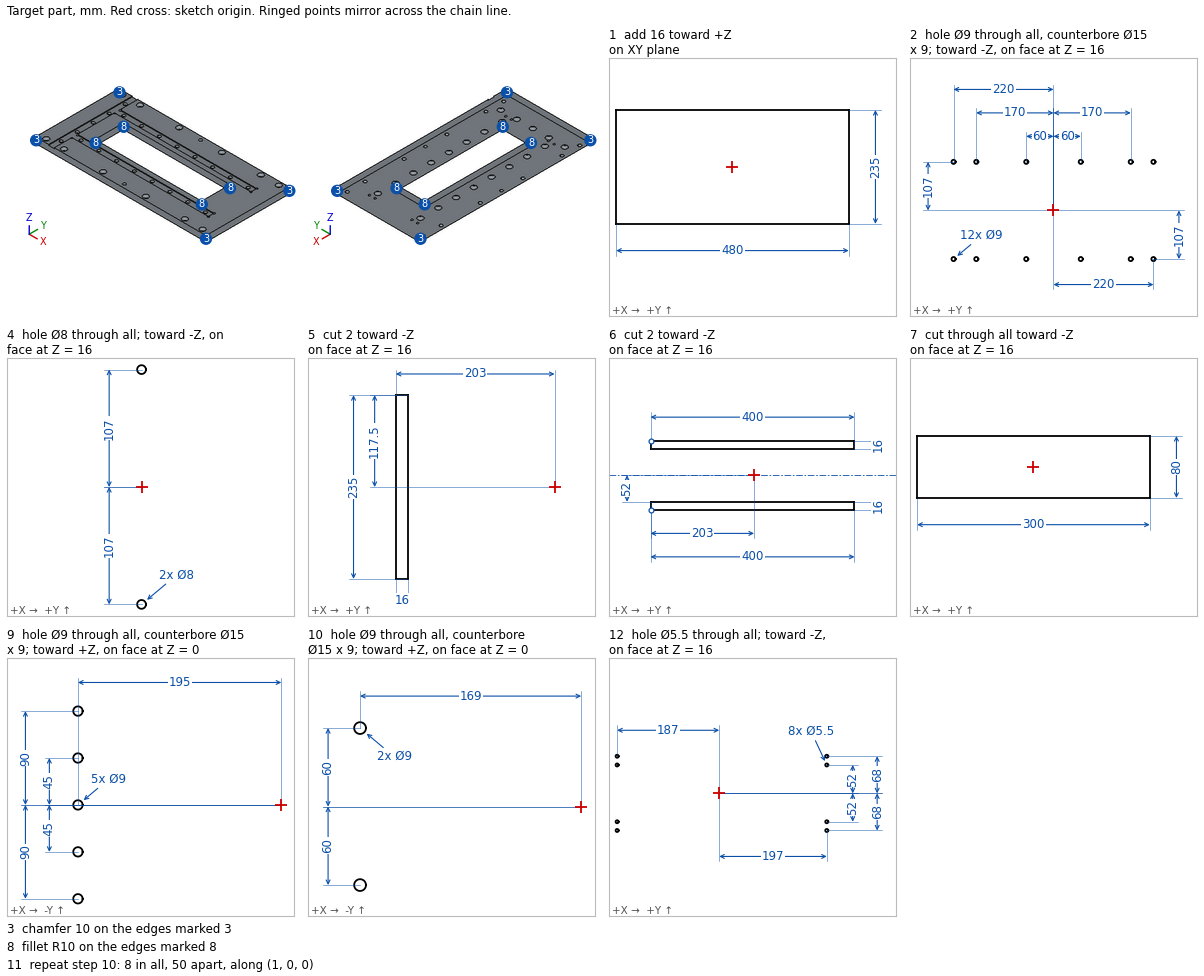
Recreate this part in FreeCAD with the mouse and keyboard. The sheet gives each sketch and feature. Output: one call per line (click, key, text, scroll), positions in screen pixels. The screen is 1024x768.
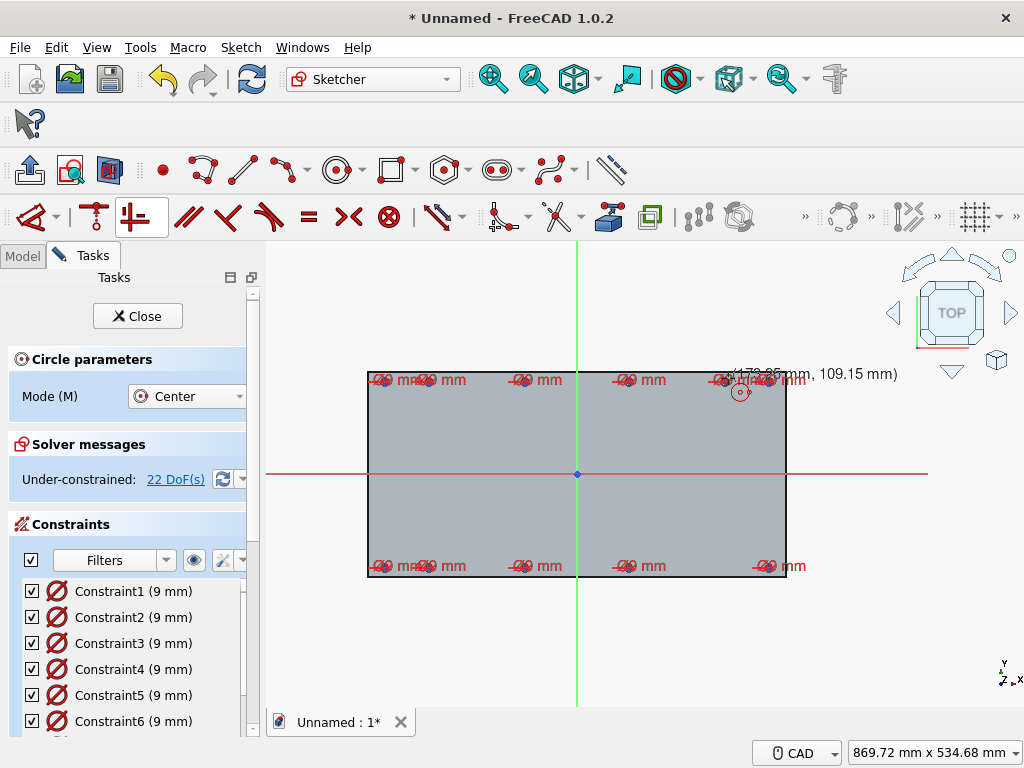
scroll(725, 567, up, 9)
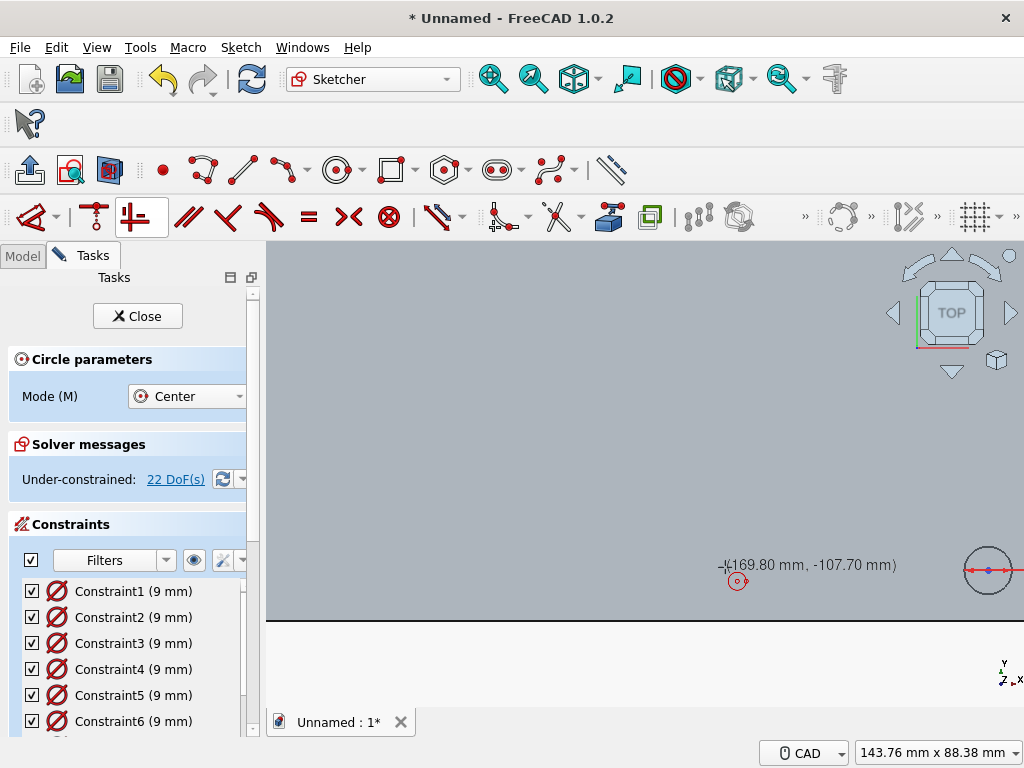
scroll(725, 568, down, 9)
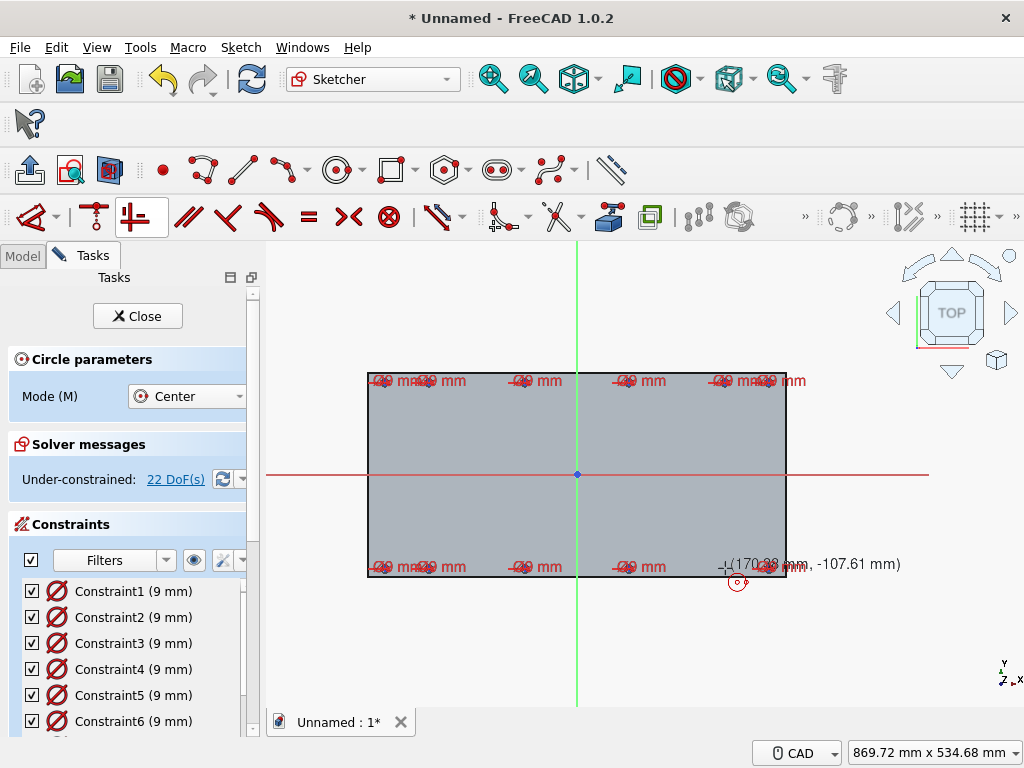
click(725, 568)
move(728, 565)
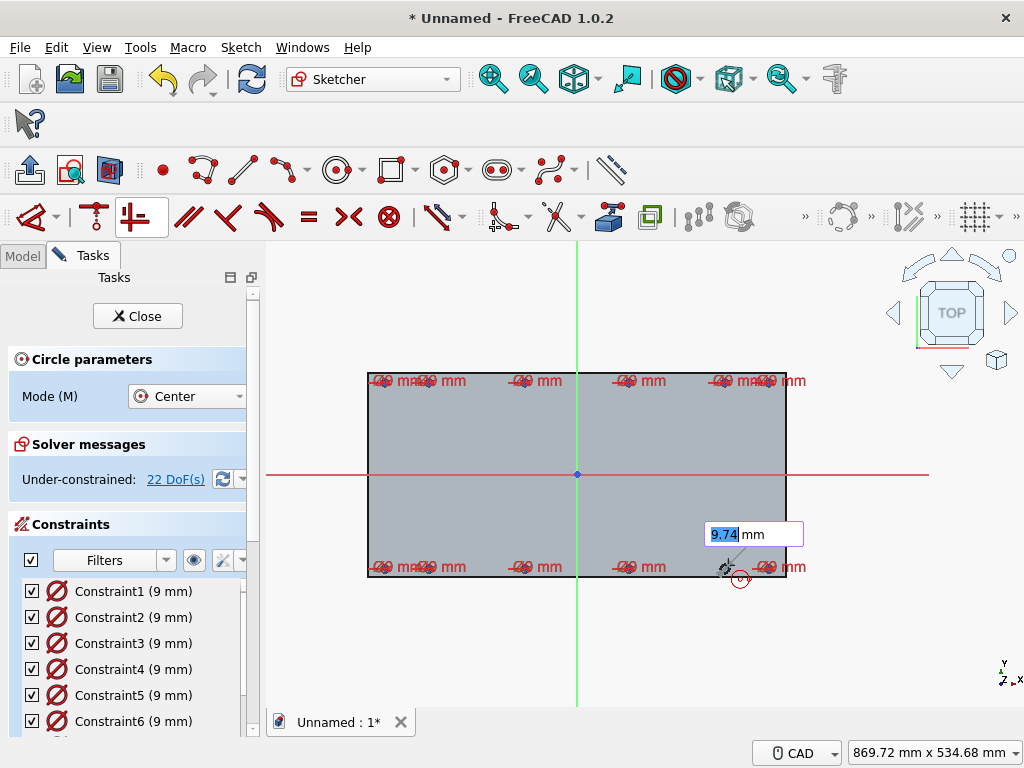
text(9)
key(Return)
key(Escape)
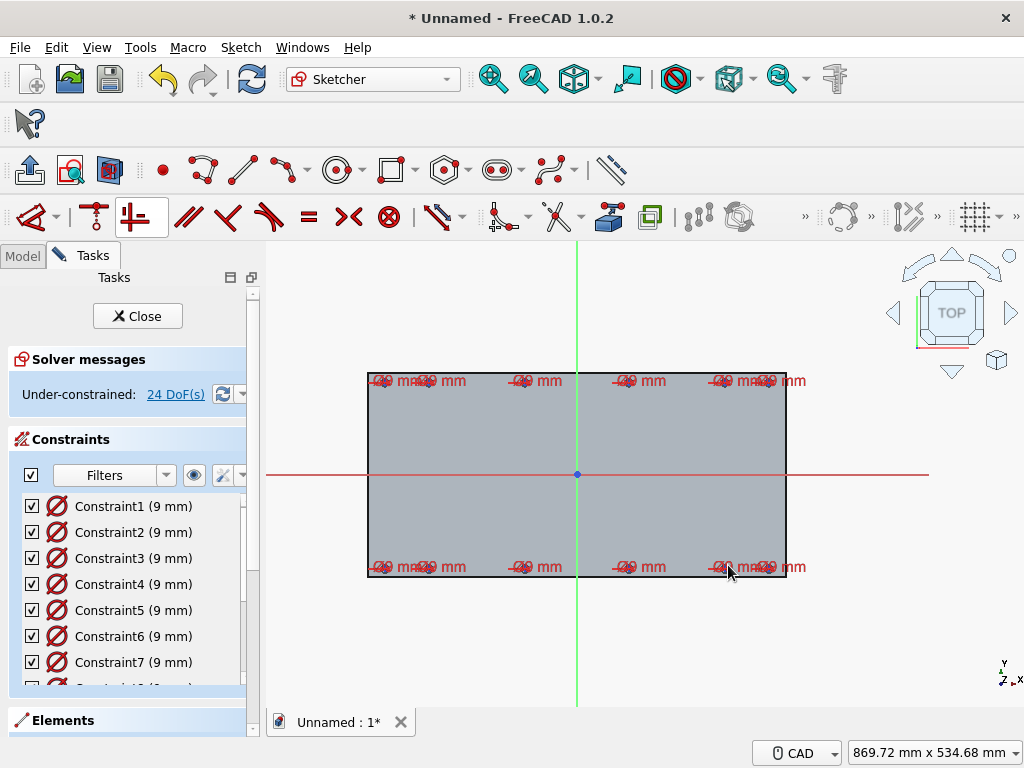
click(385, 383)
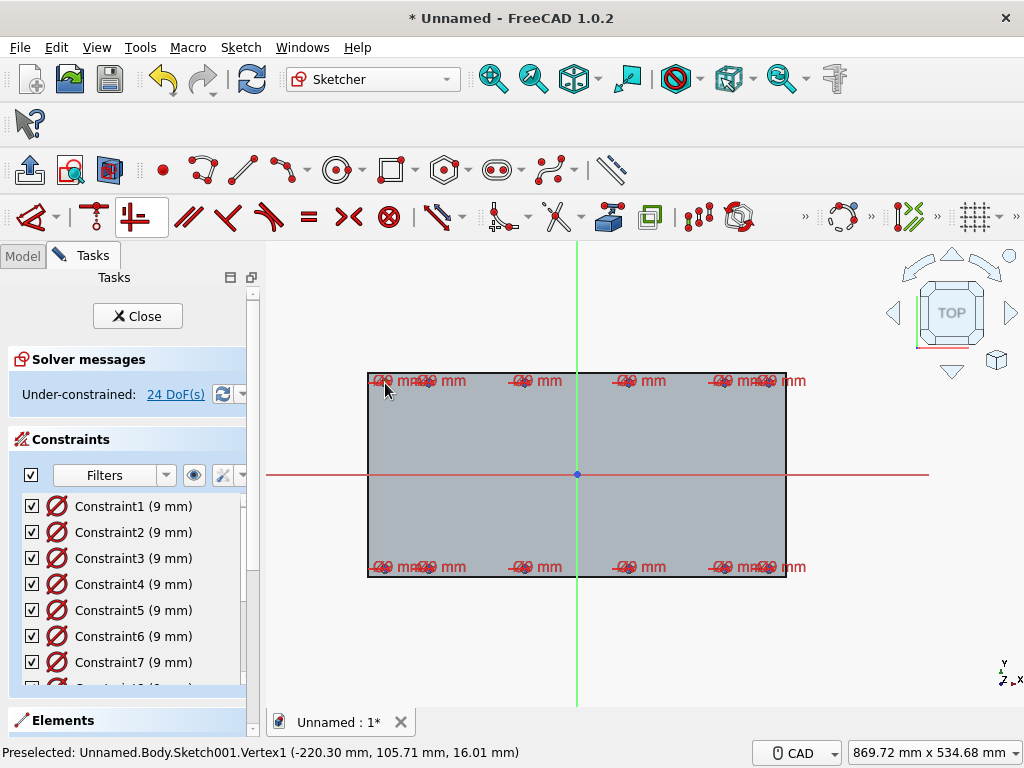
click(385, 569)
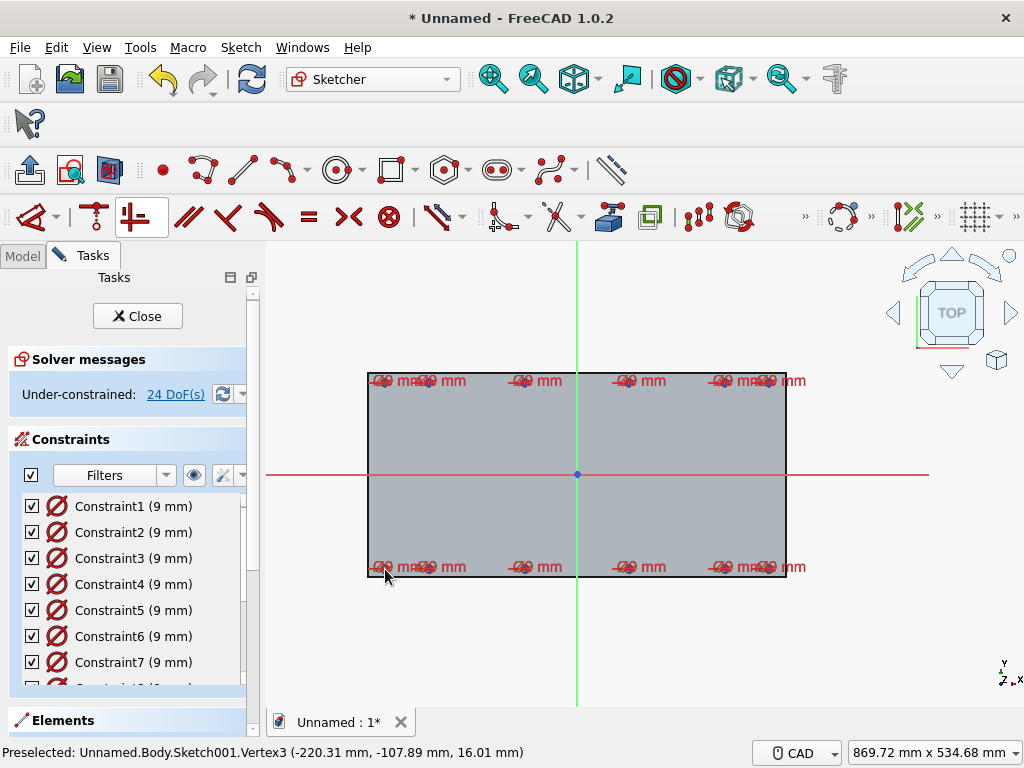
click(162, 218)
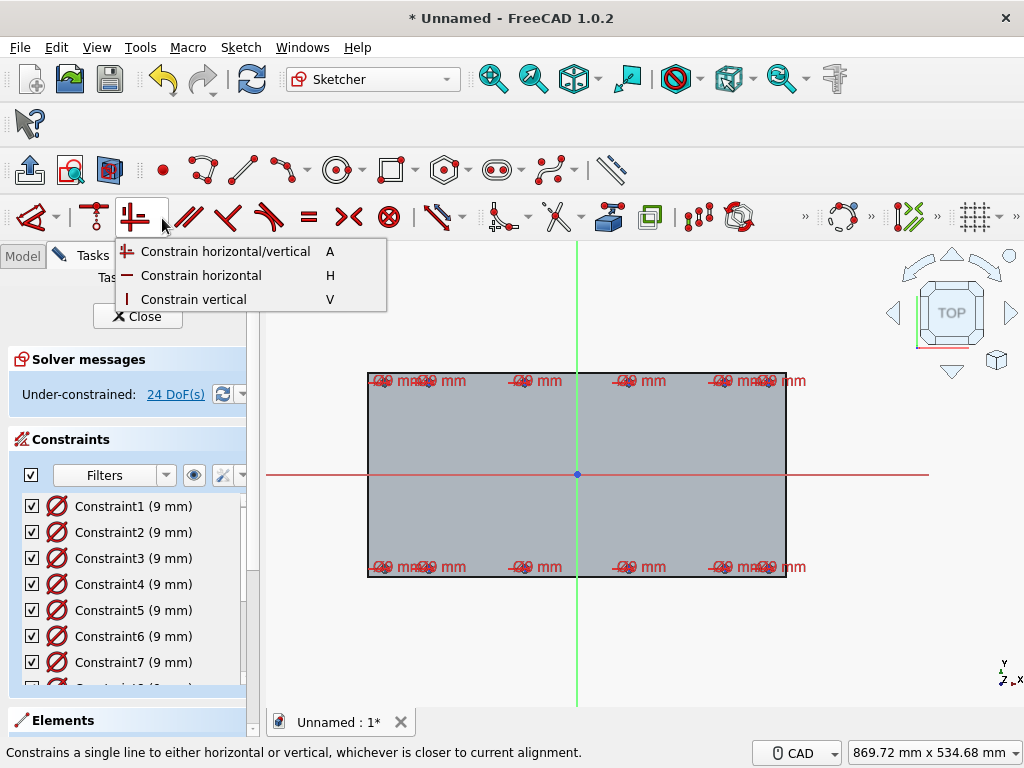
click(251, 299)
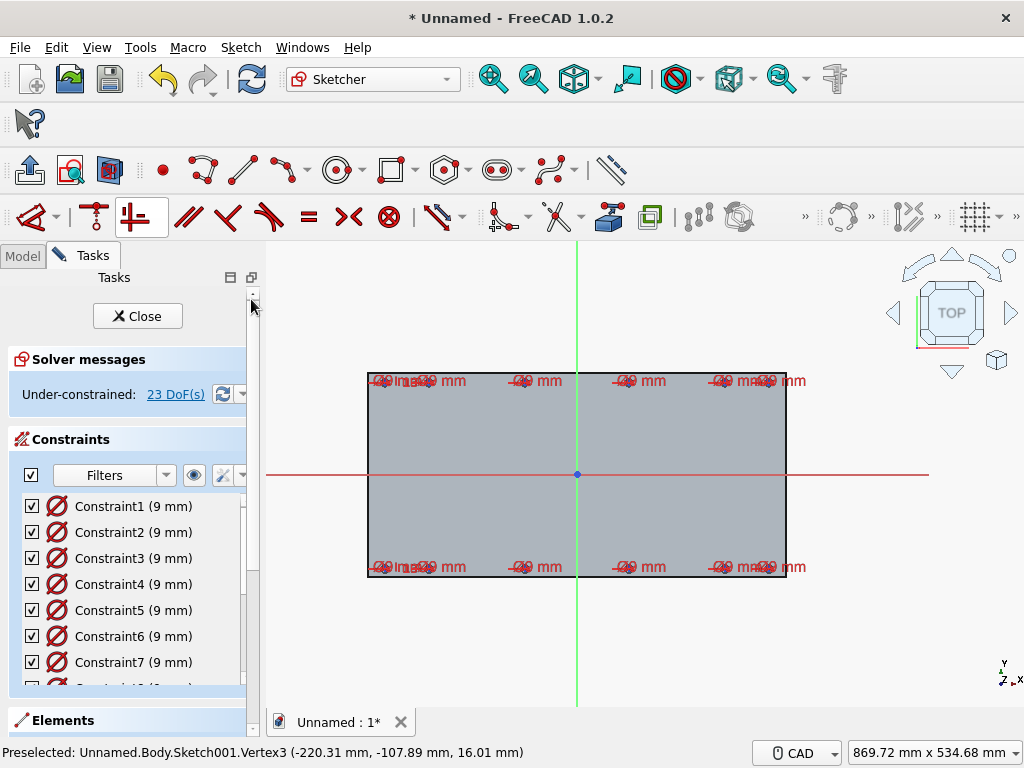
click(769, 569)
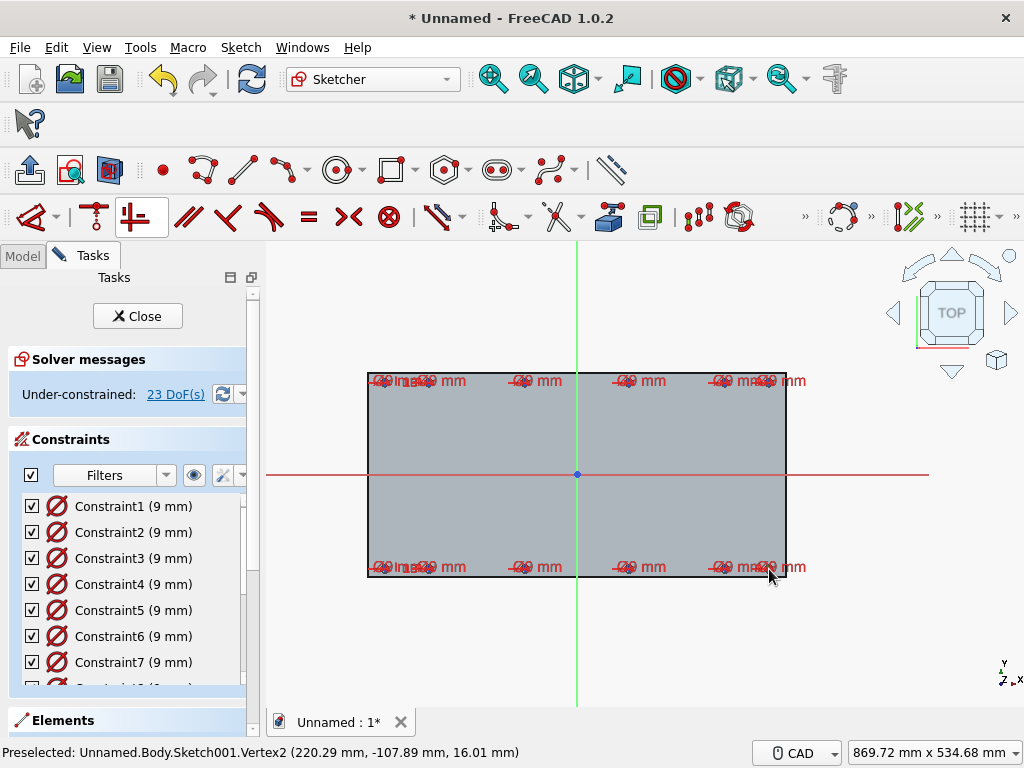
click(385, 569)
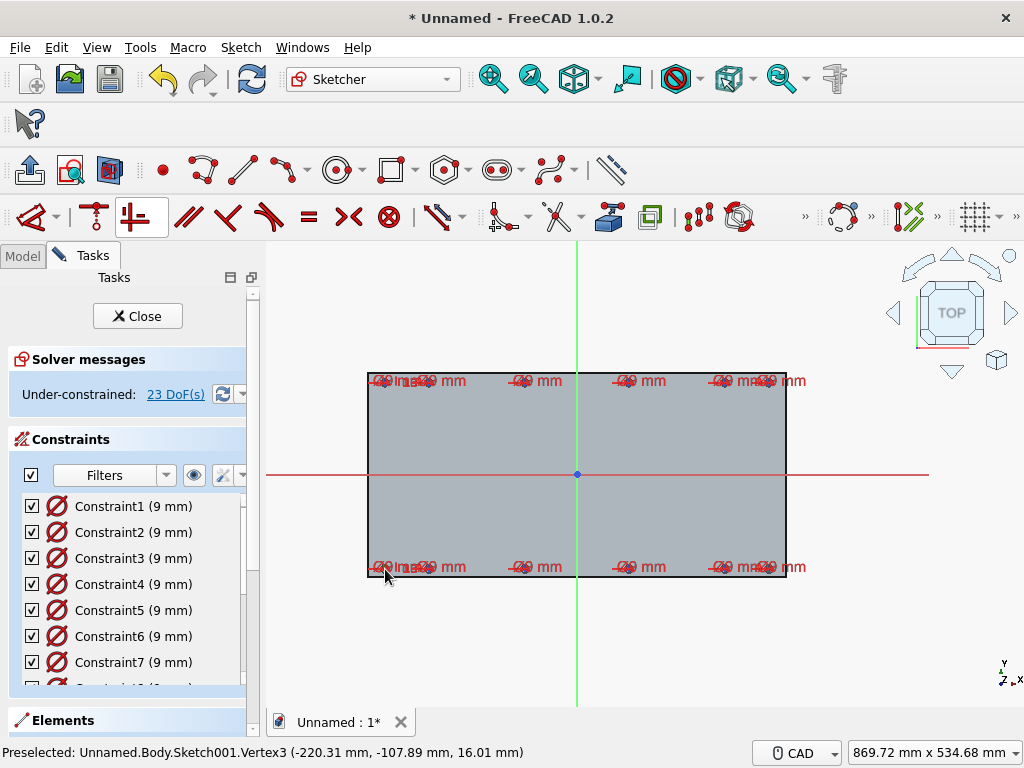
key(h)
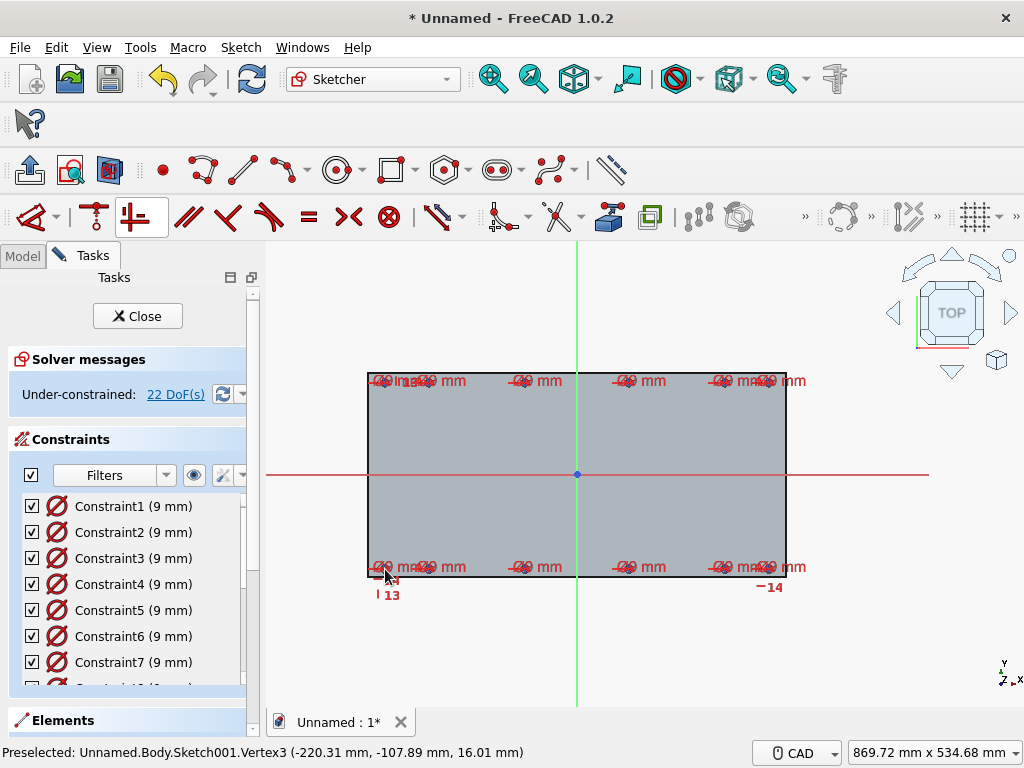
click(769, 569)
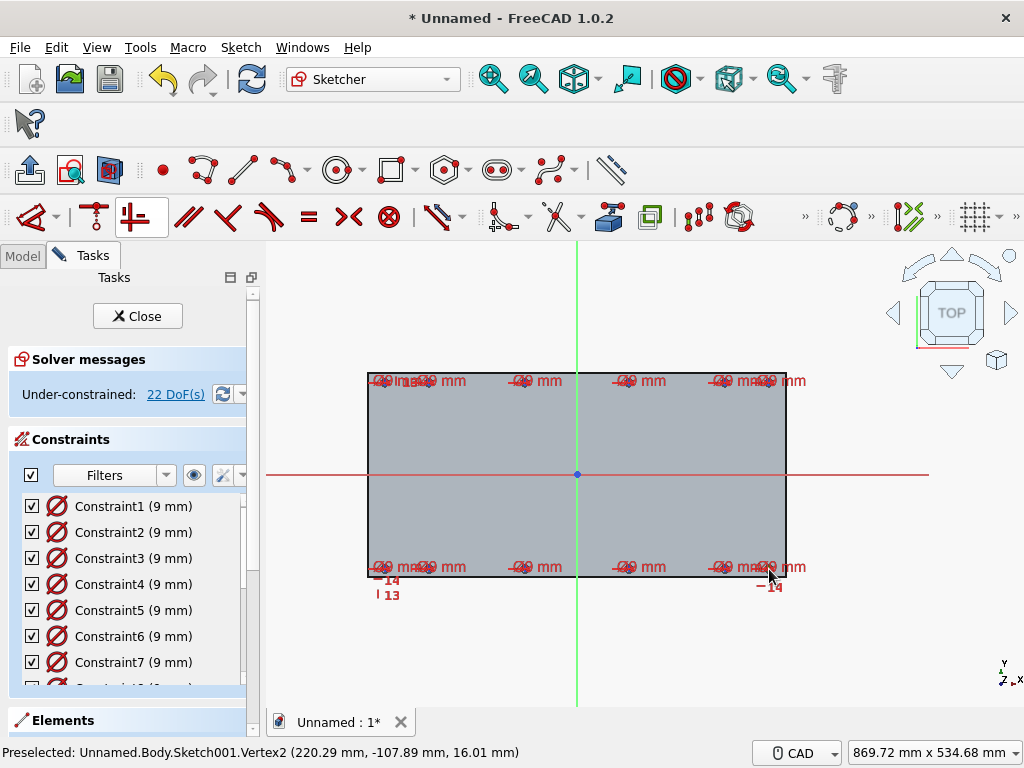
click(769, 383)